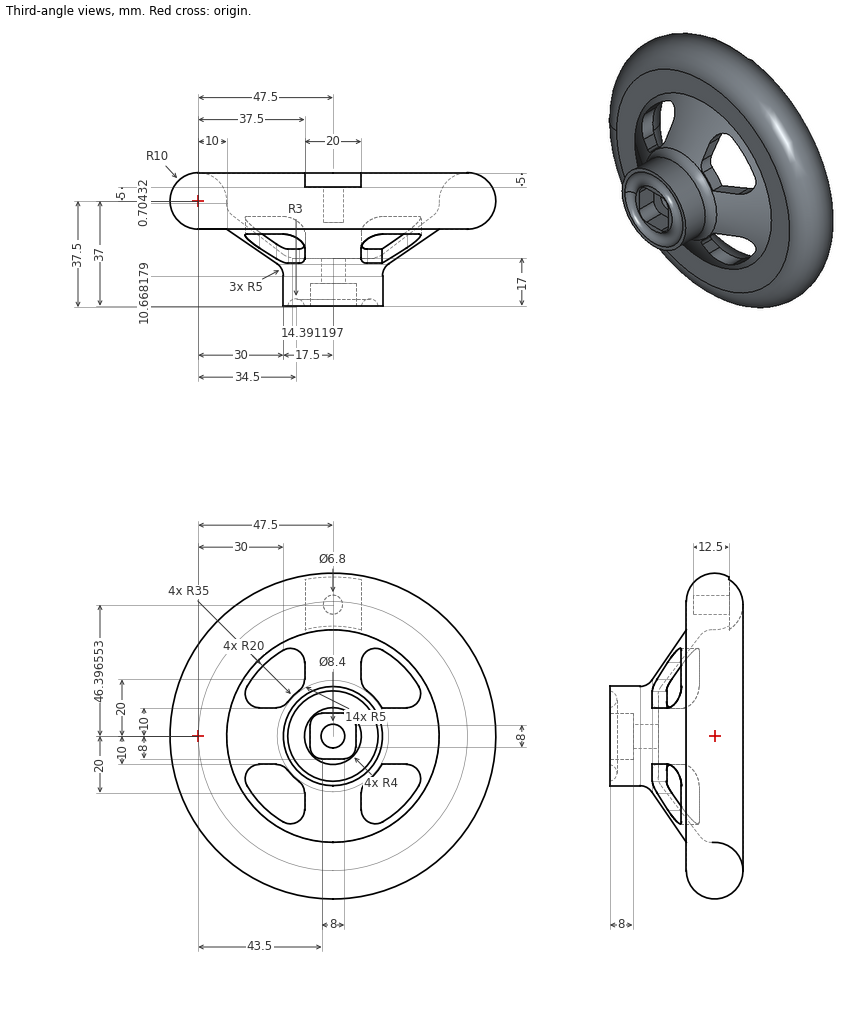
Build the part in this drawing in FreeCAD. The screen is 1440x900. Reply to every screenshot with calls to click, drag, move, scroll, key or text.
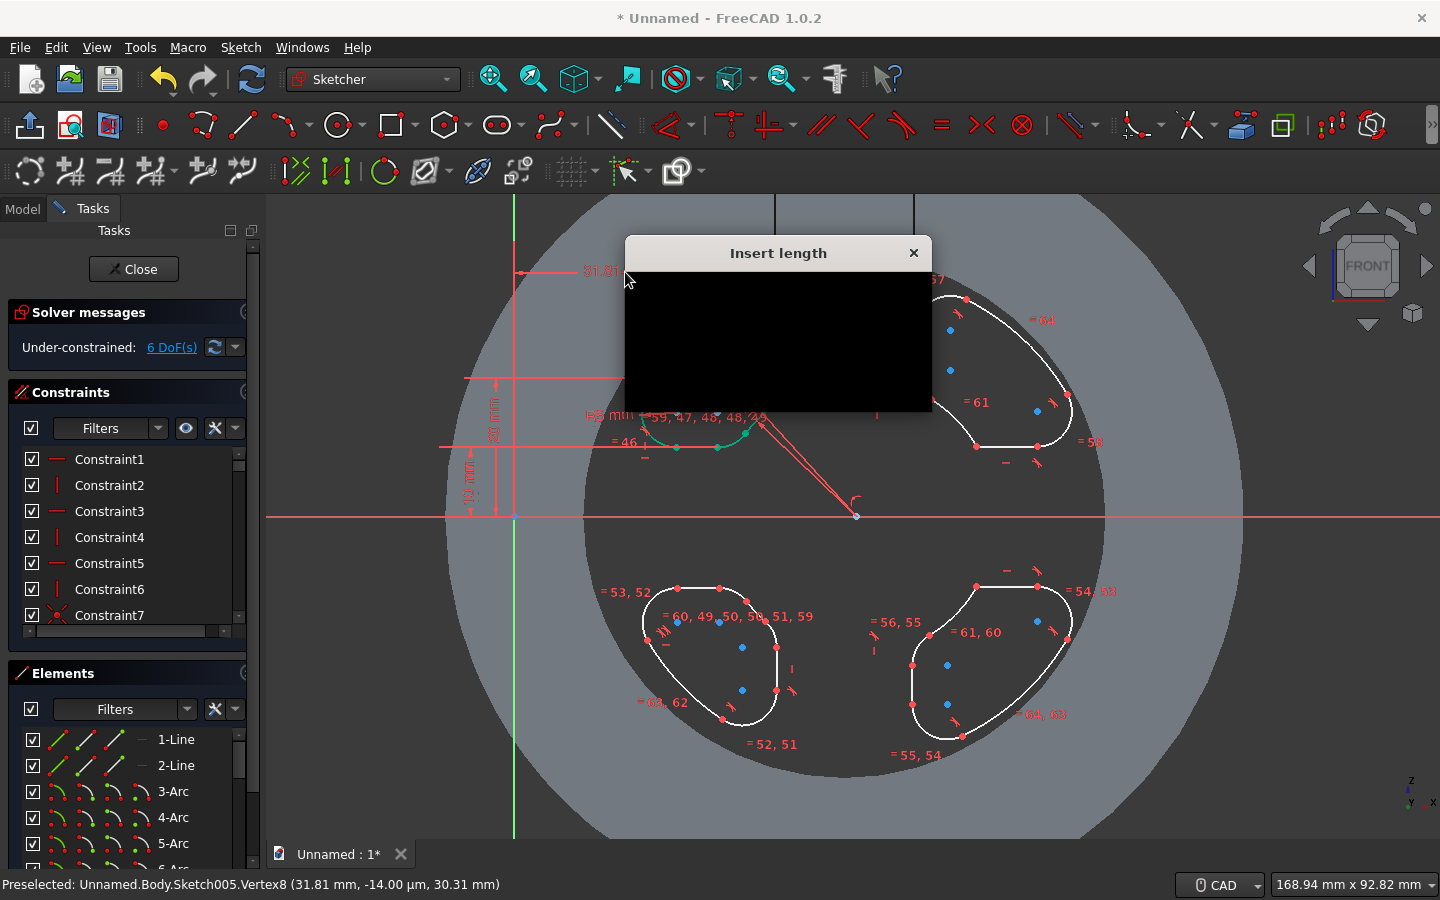
text(30)
key(Return)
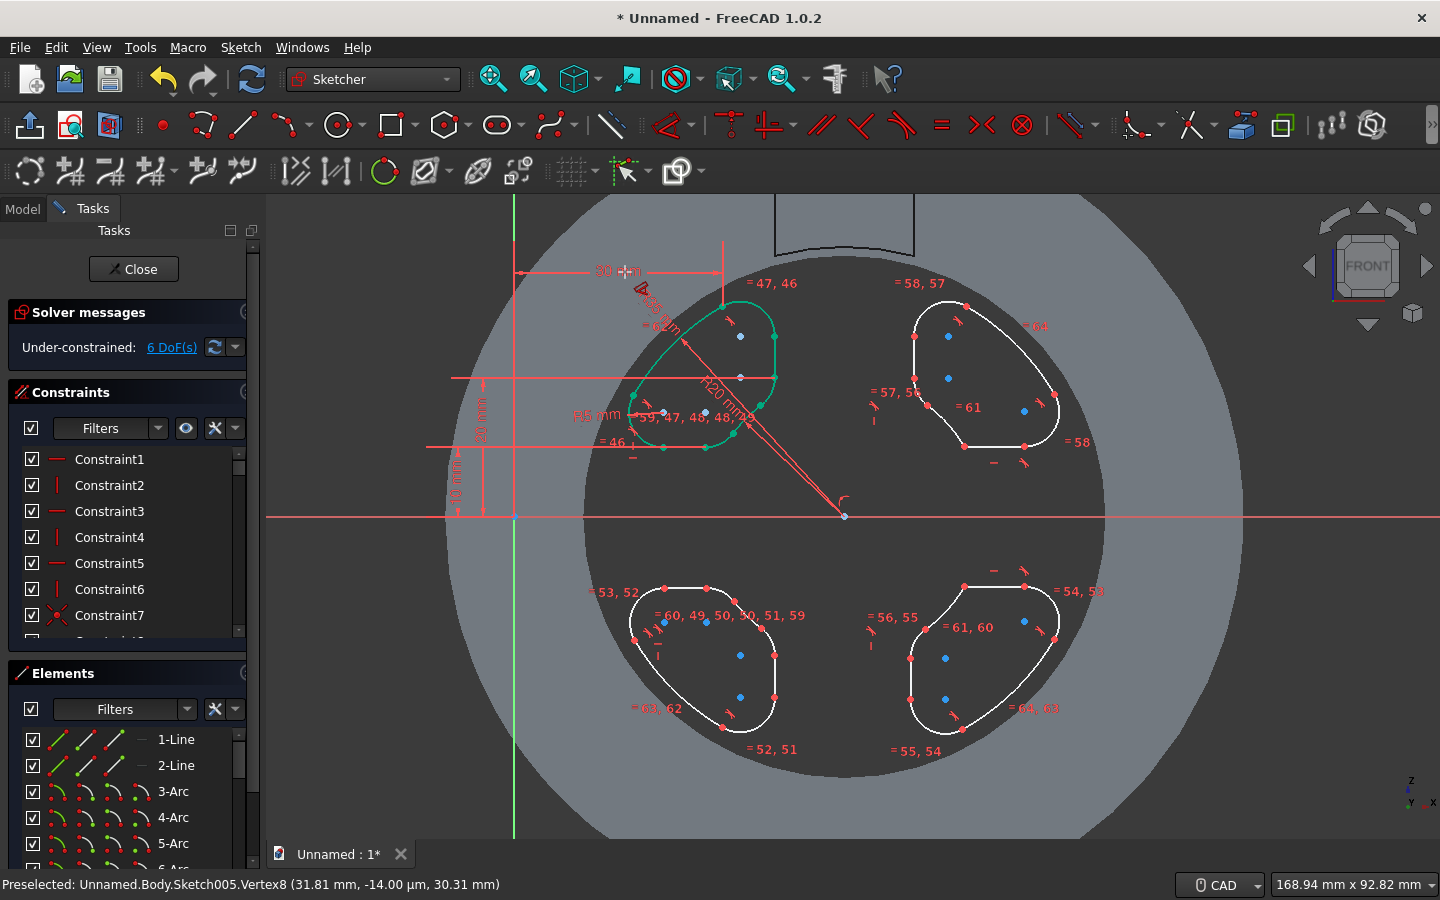
click(665, 588)
click(480, 552)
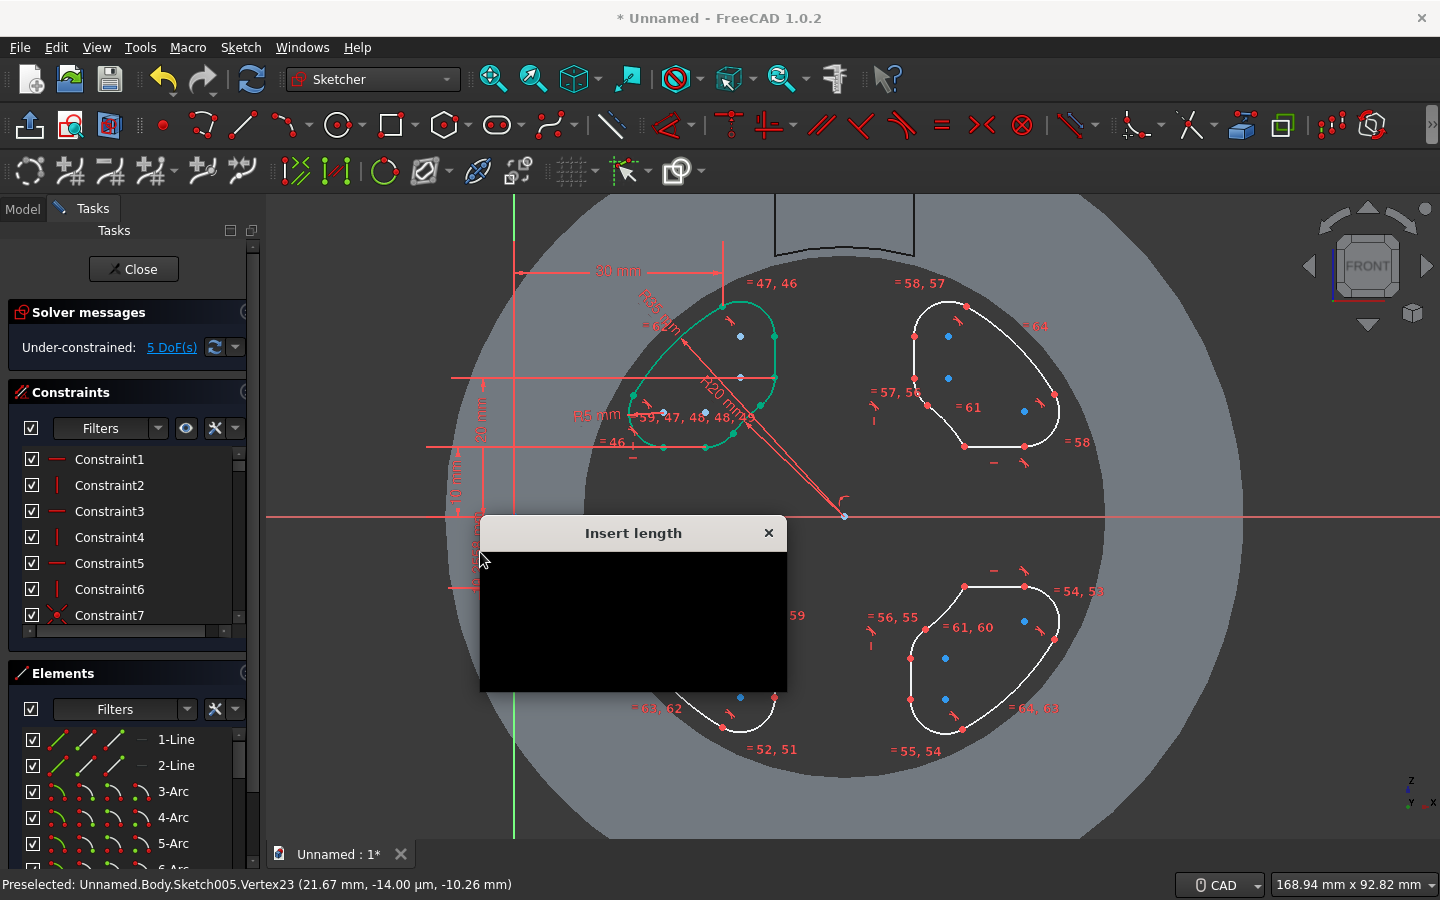
text(10)
key(Return)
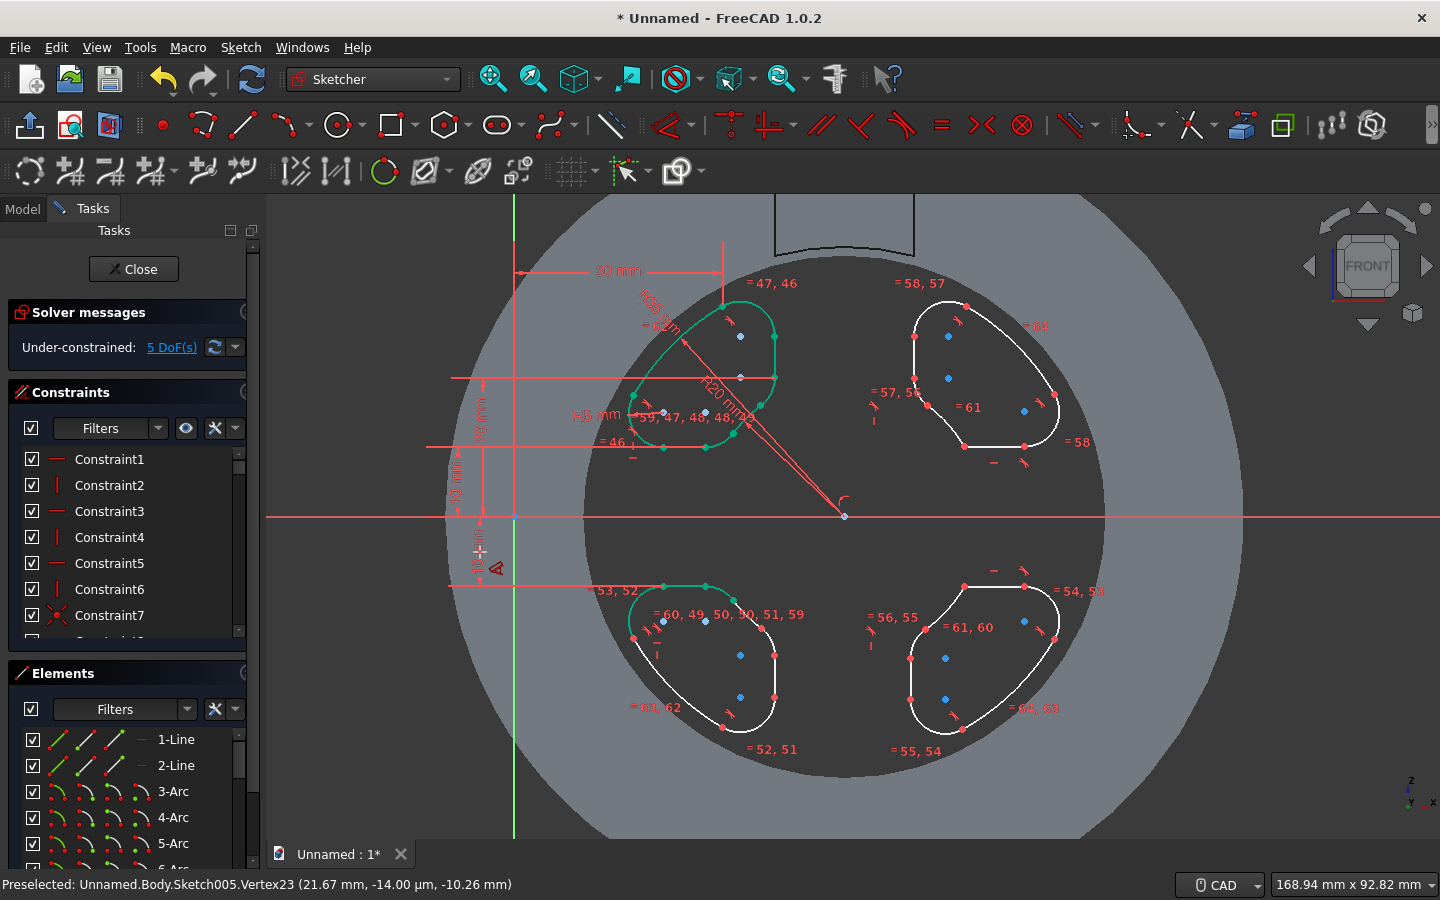
click(775, 656)
click(480, 586)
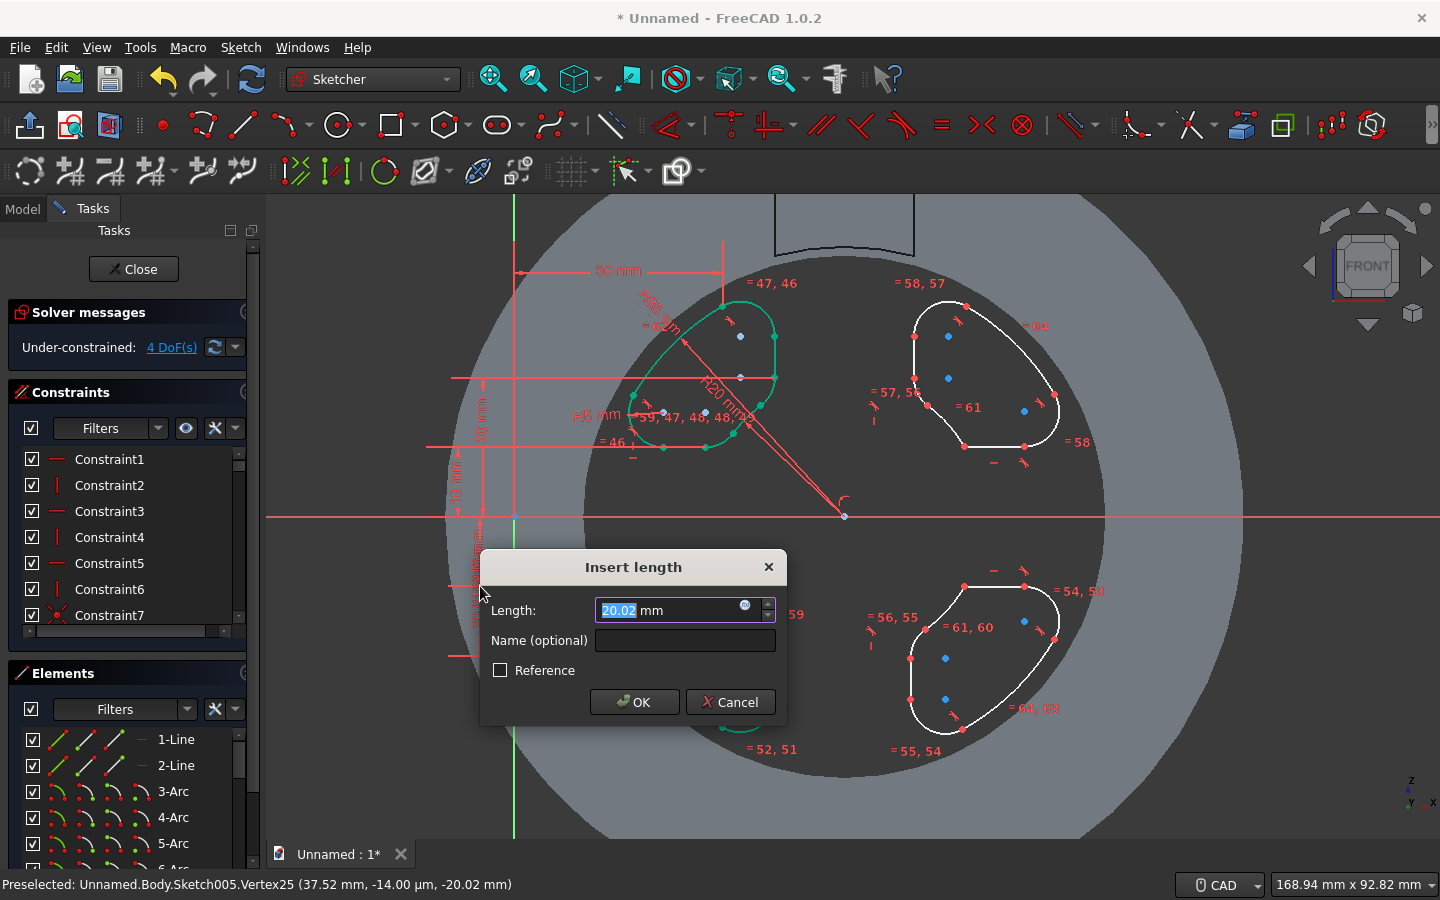
text(20)
key(Return)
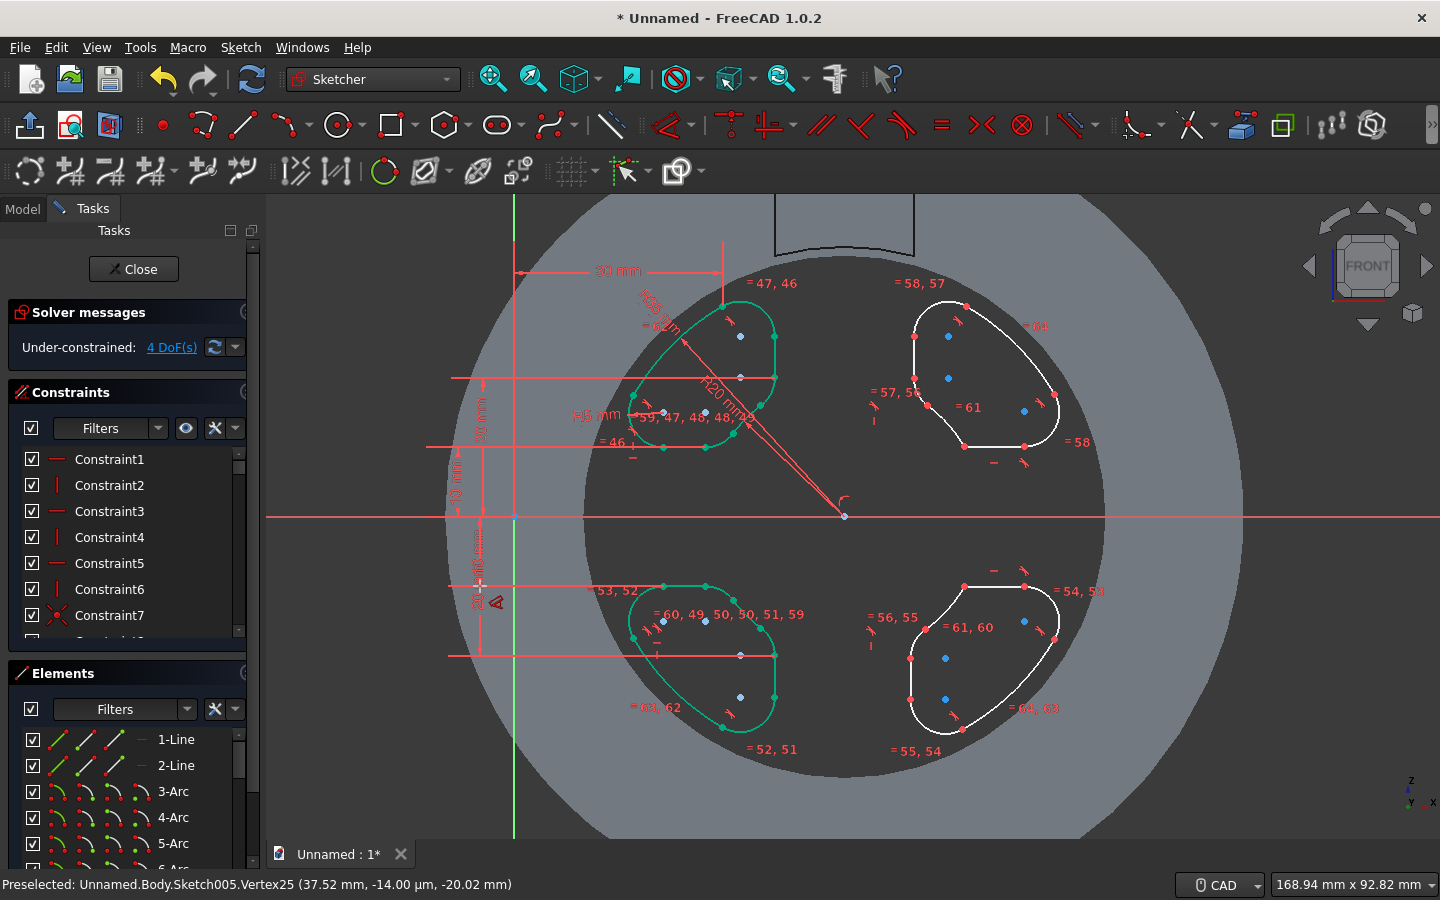
click(964, 587)
click(998, 552)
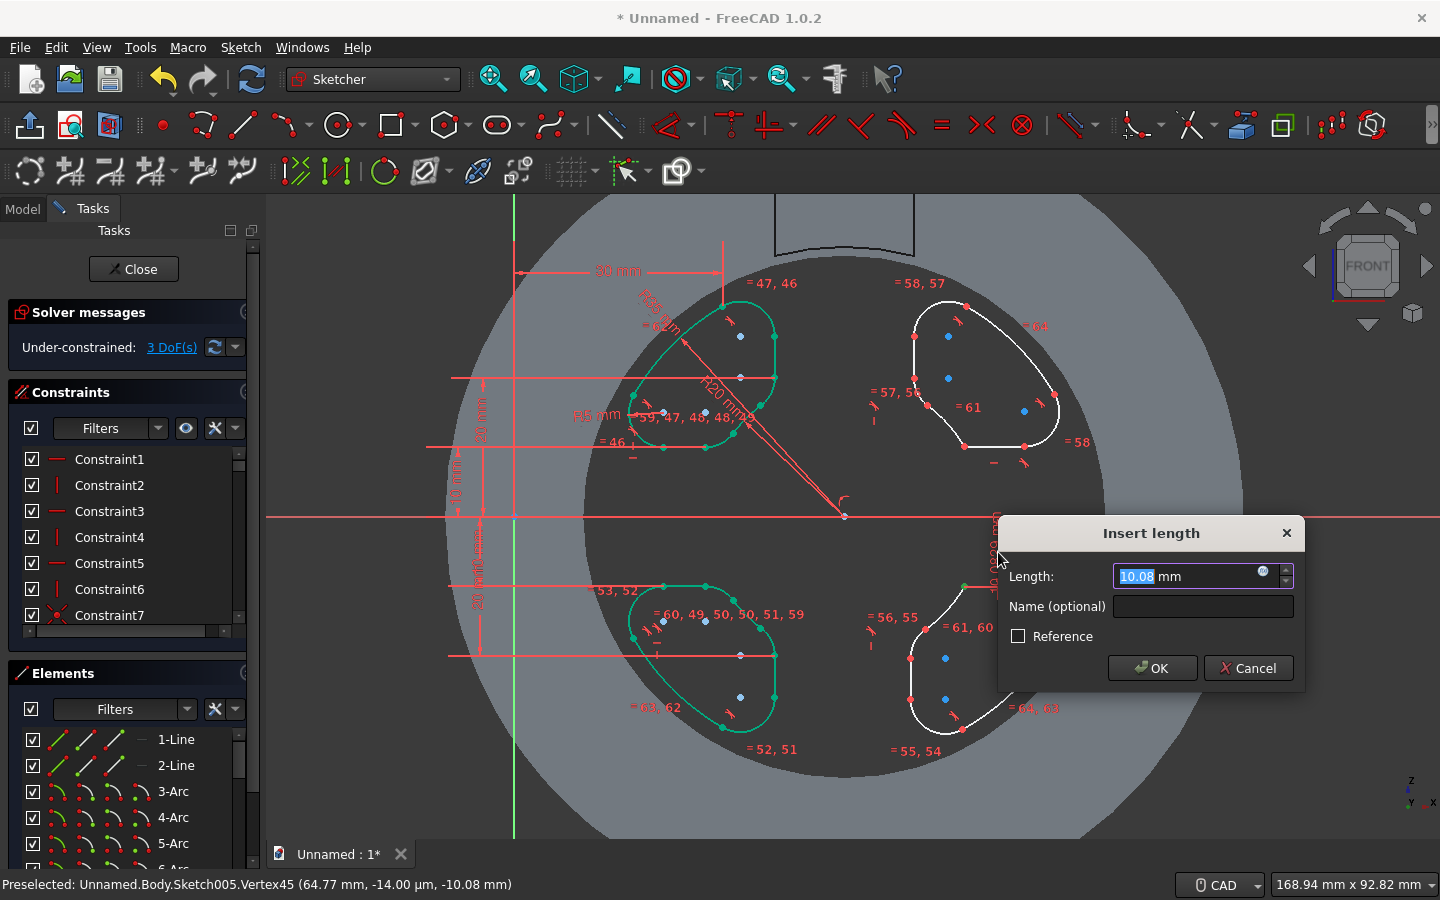
text(10)
key(Return)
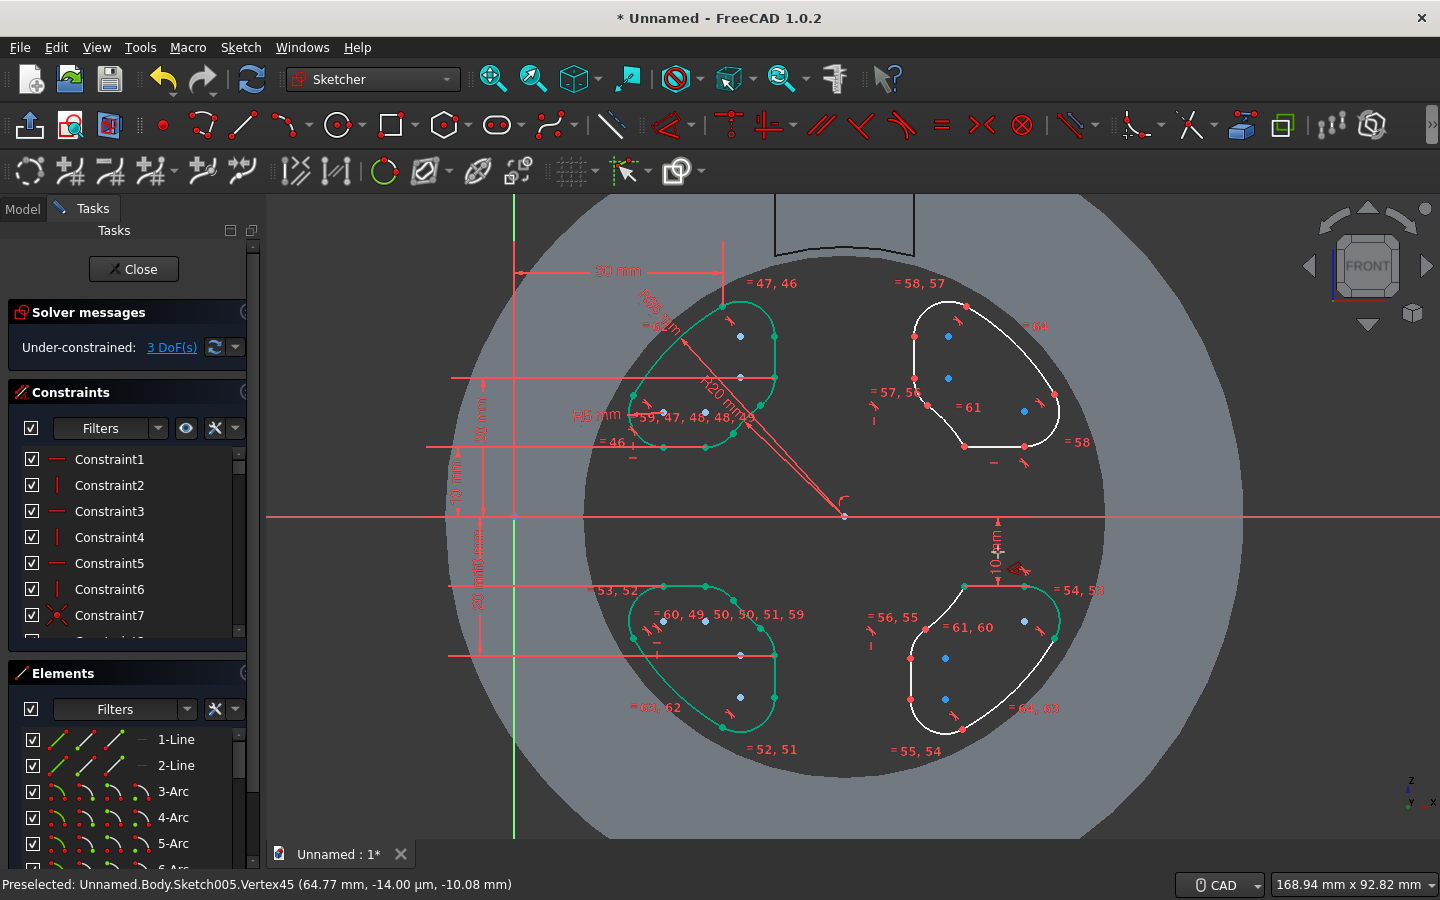
click(911, 658)
click(480, 620)